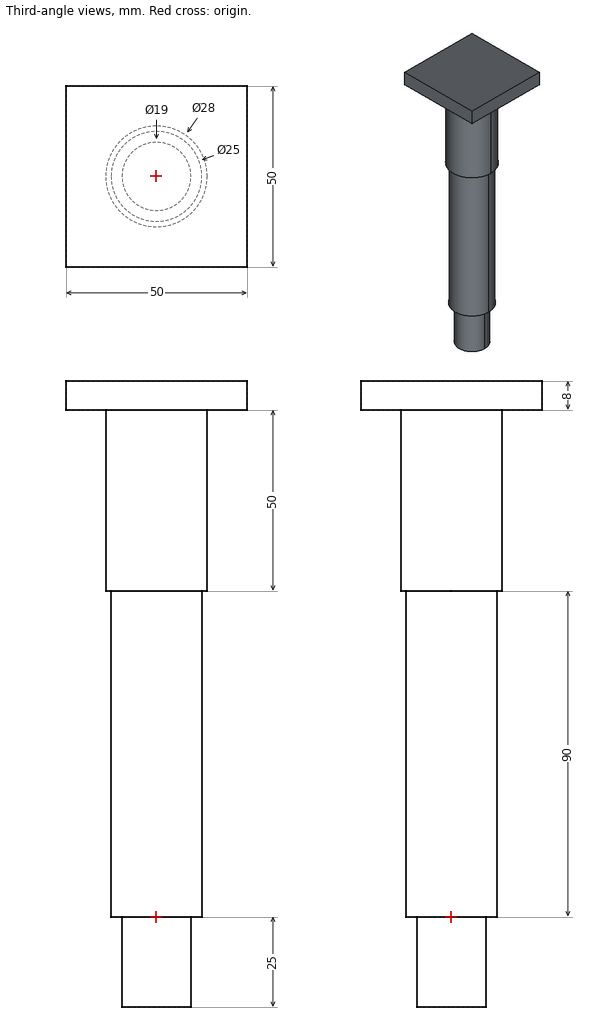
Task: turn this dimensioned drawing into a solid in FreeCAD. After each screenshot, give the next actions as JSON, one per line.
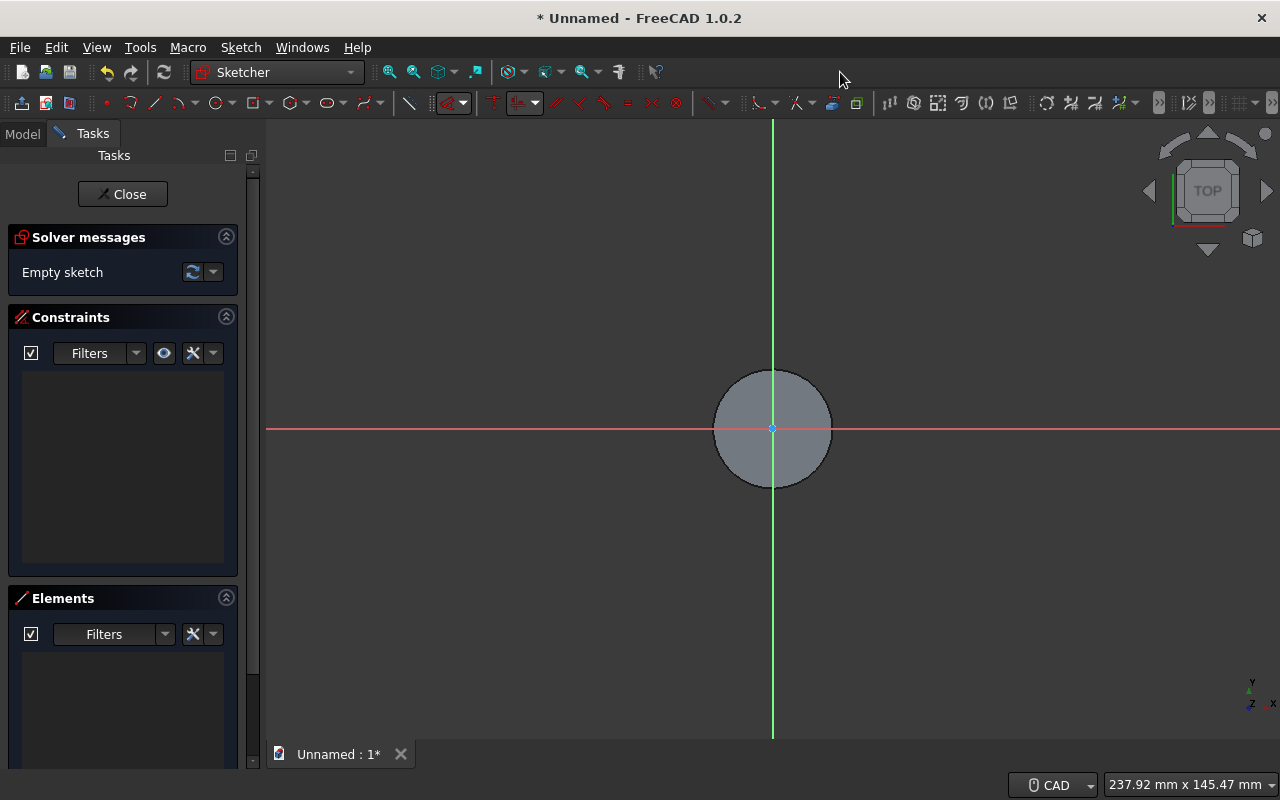
{"action": "scroll", "coordinate": [856, 429], "scroll_direction": "up", "scroll_amount": 3}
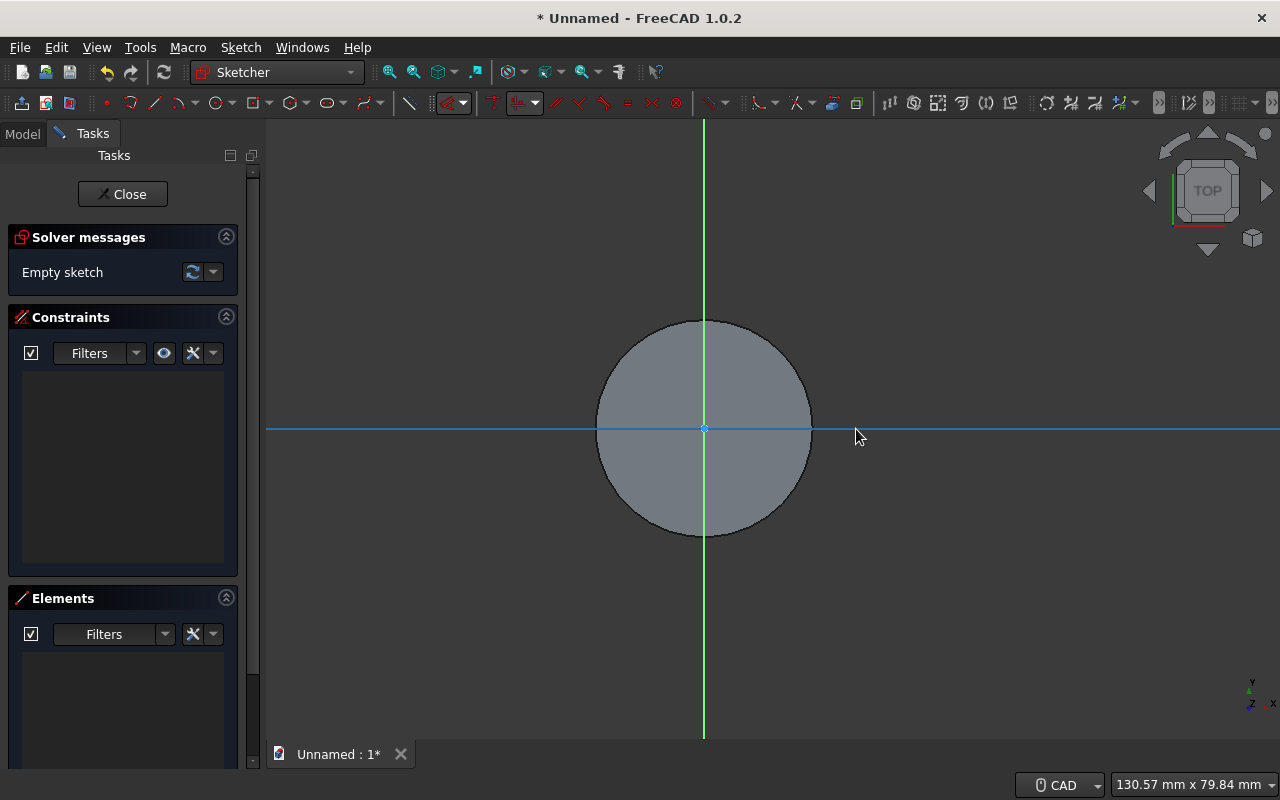
{"action": "key", "text": "g v"}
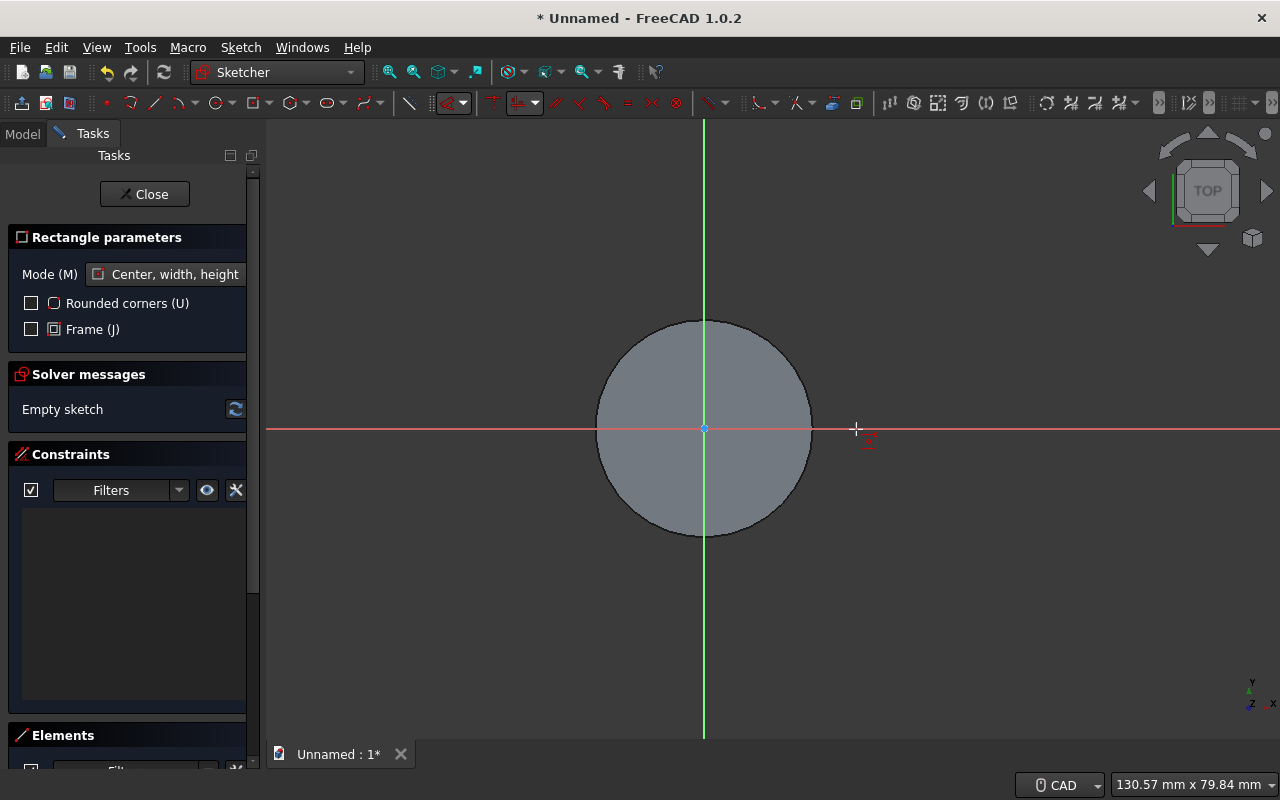
{"action": "left_click", "coordinate": [704, 429]}
{"action": "left_click", "coordinate": [898, 234]}
{"action": "key", "text": "Escape"}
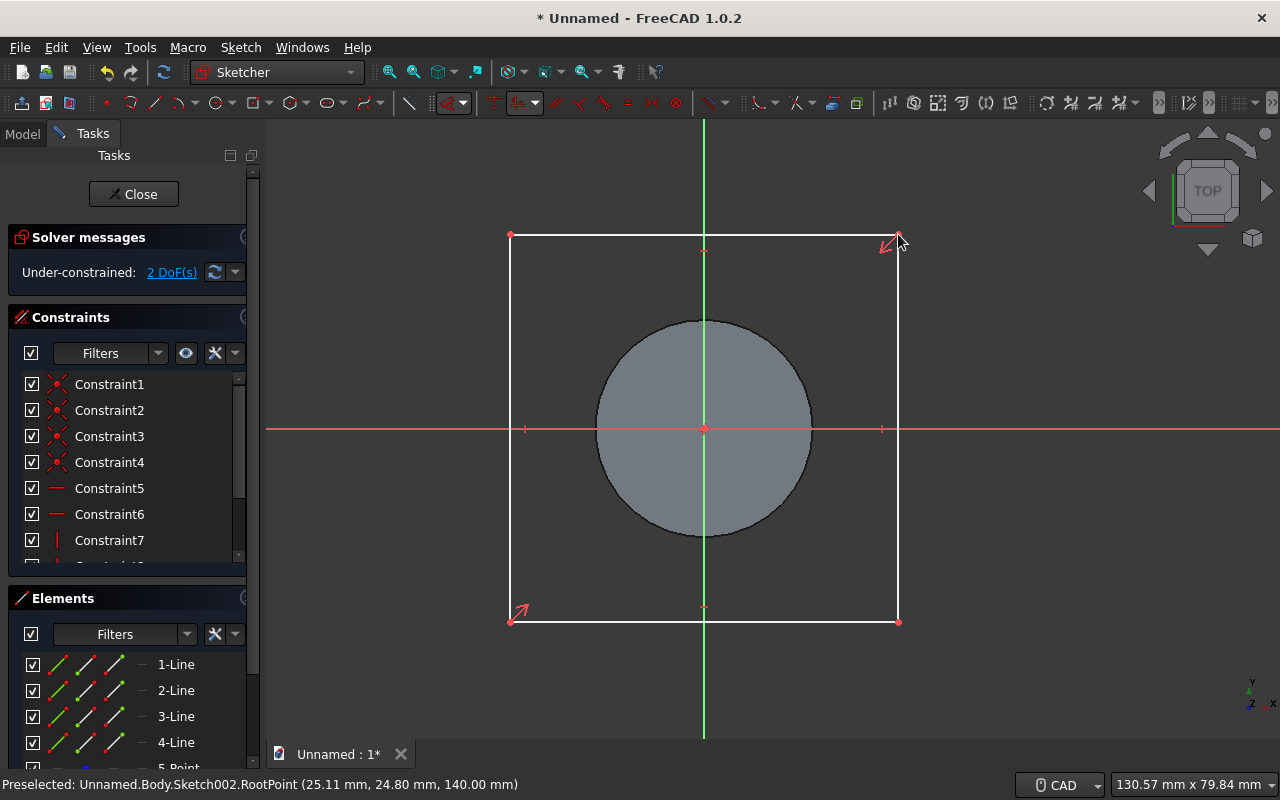
{"action": "left_click", "coordinate": [448, 104]}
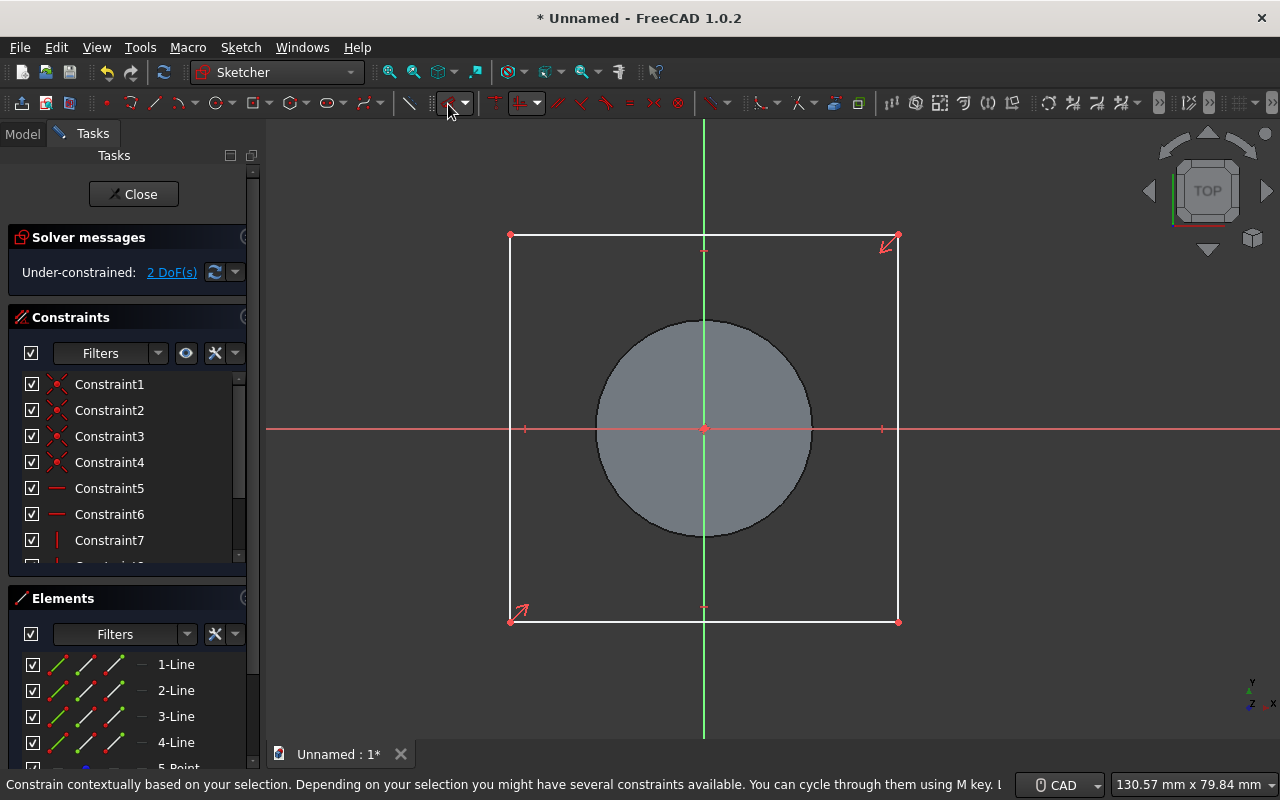
{"action": "left_click", "coordinate": [626, 622]}
{"action": "left_click", "coordinate": [615, 656]}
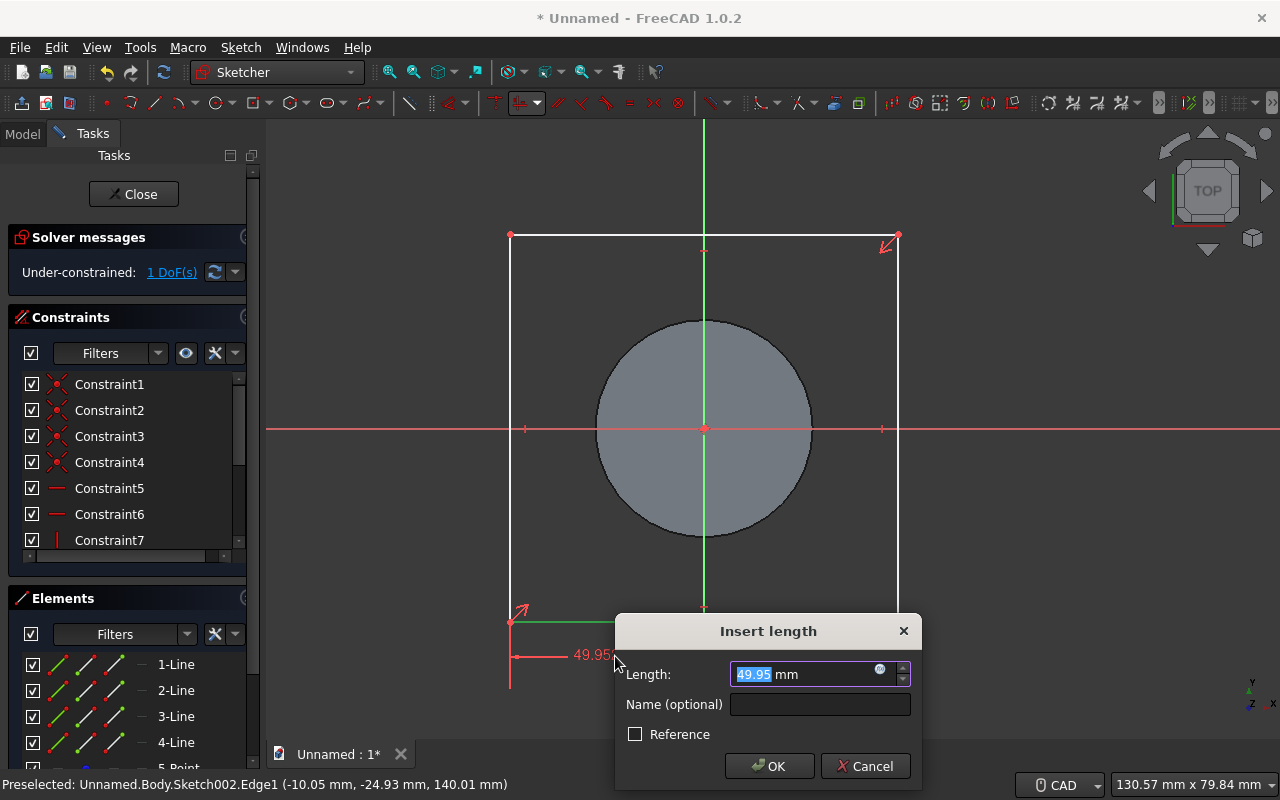
{"action": "type", "text": "50"}
{"action": "key", "text": "Return"}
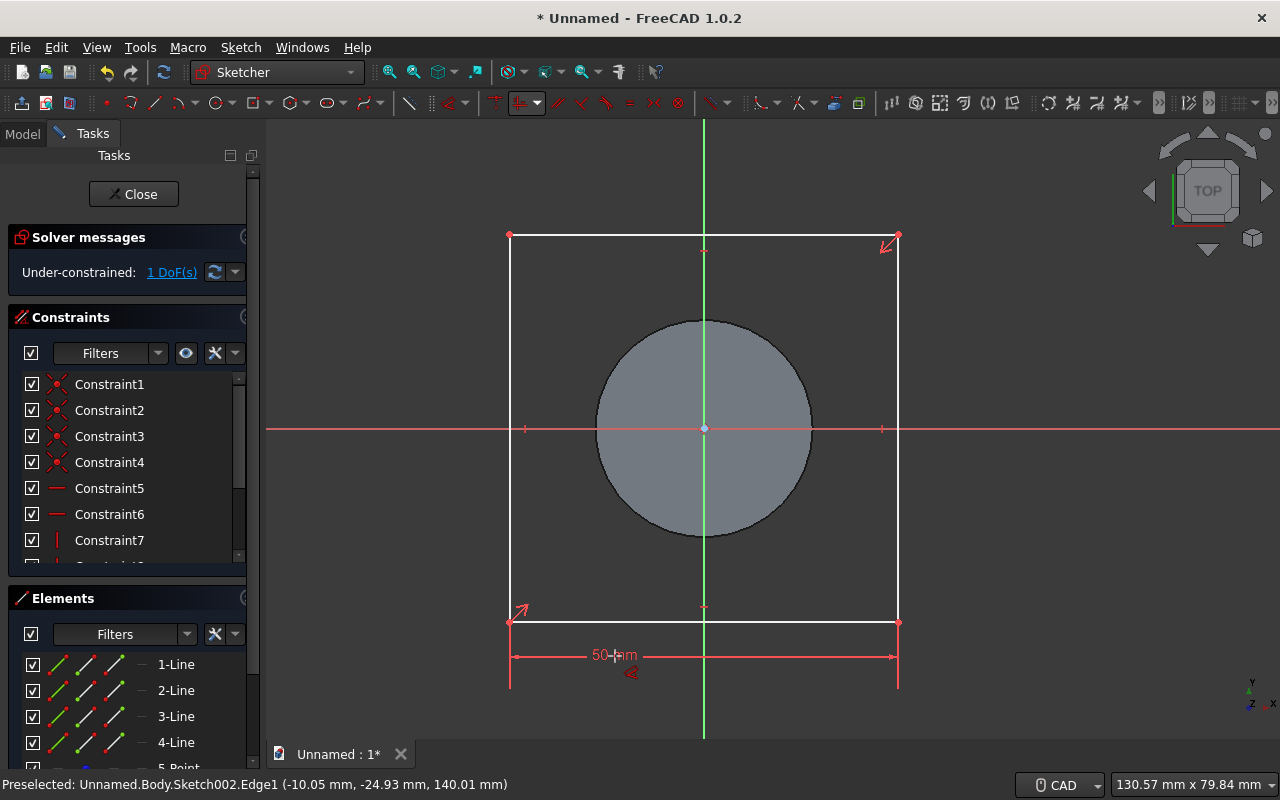
{"action": "left_click", "coordinate": [898, 506]}
{"action": "left_click", "coordinate": [932, 340]}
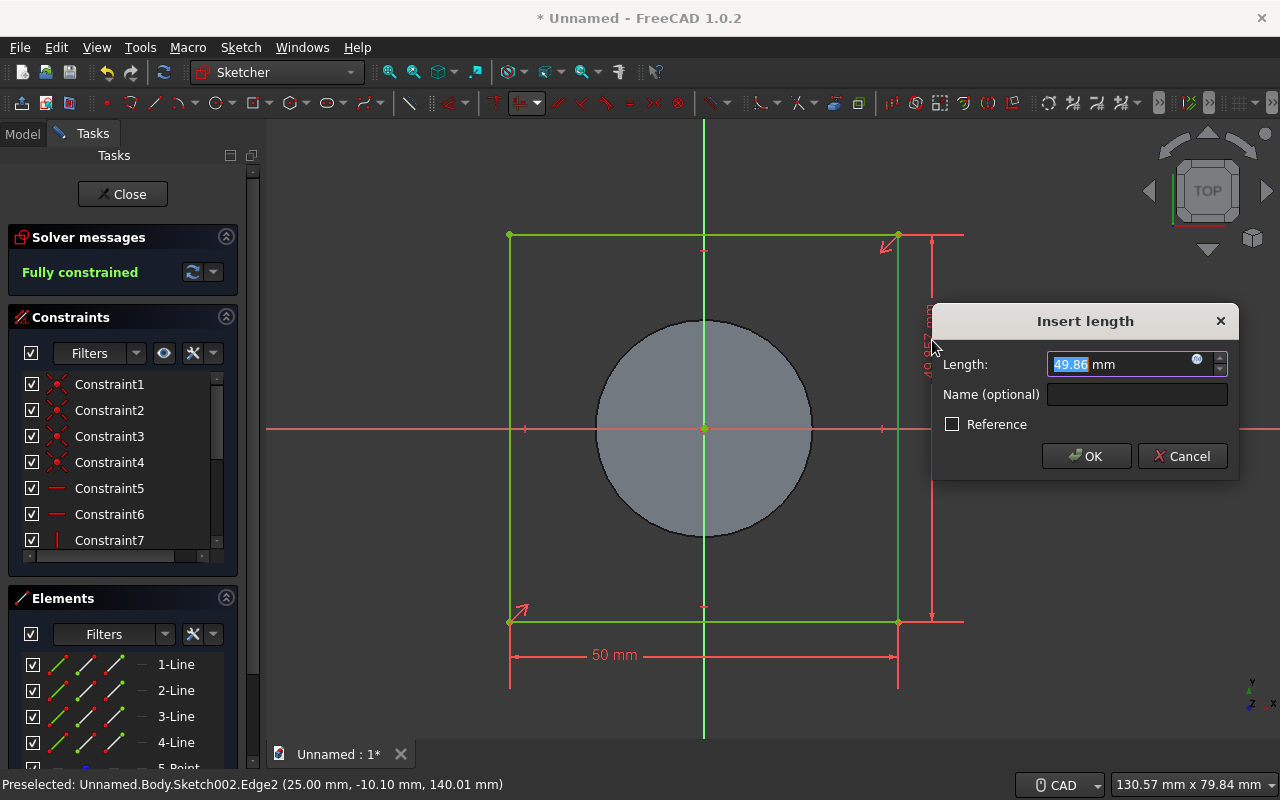
{"action": "type", "text": "50"}
{"action": "key", "text": "Return"}
{"action": "key", "text": "Escape"}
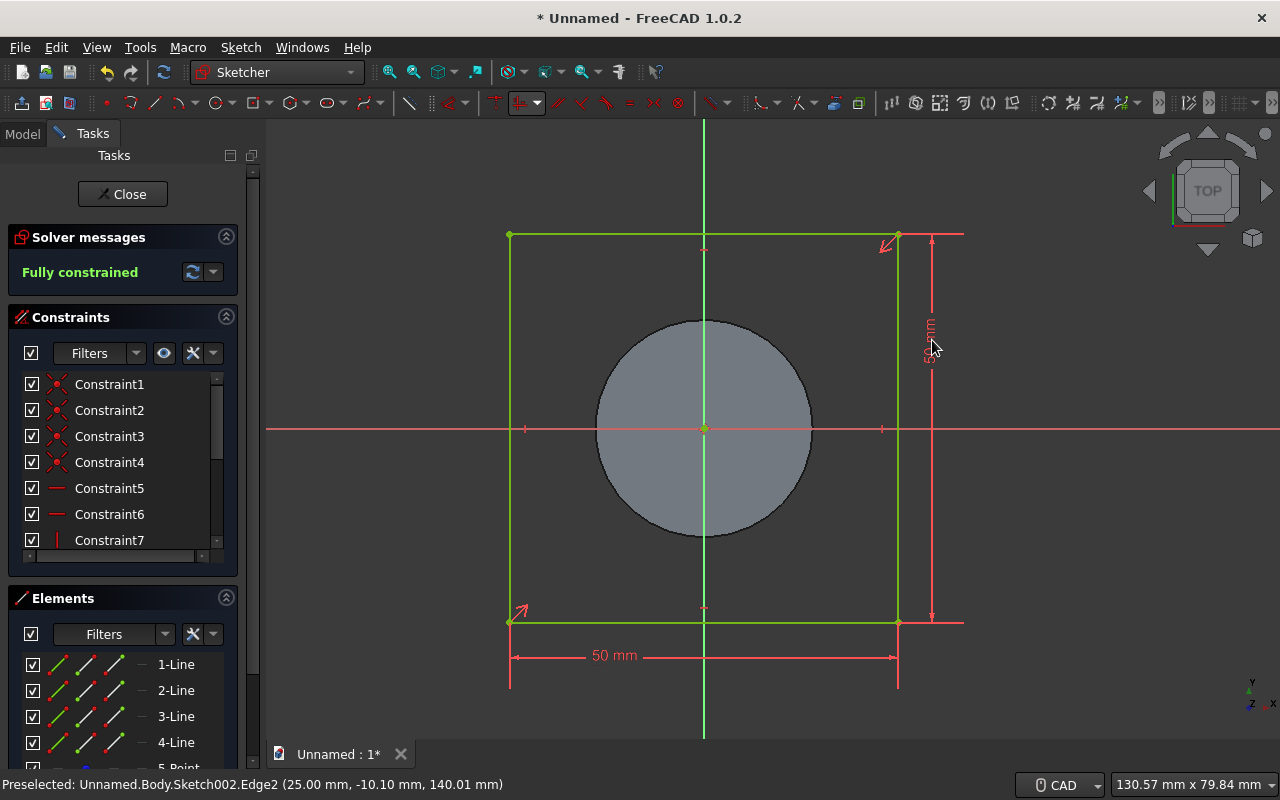
{"action": "left_click", "coordinate": [123, 194]}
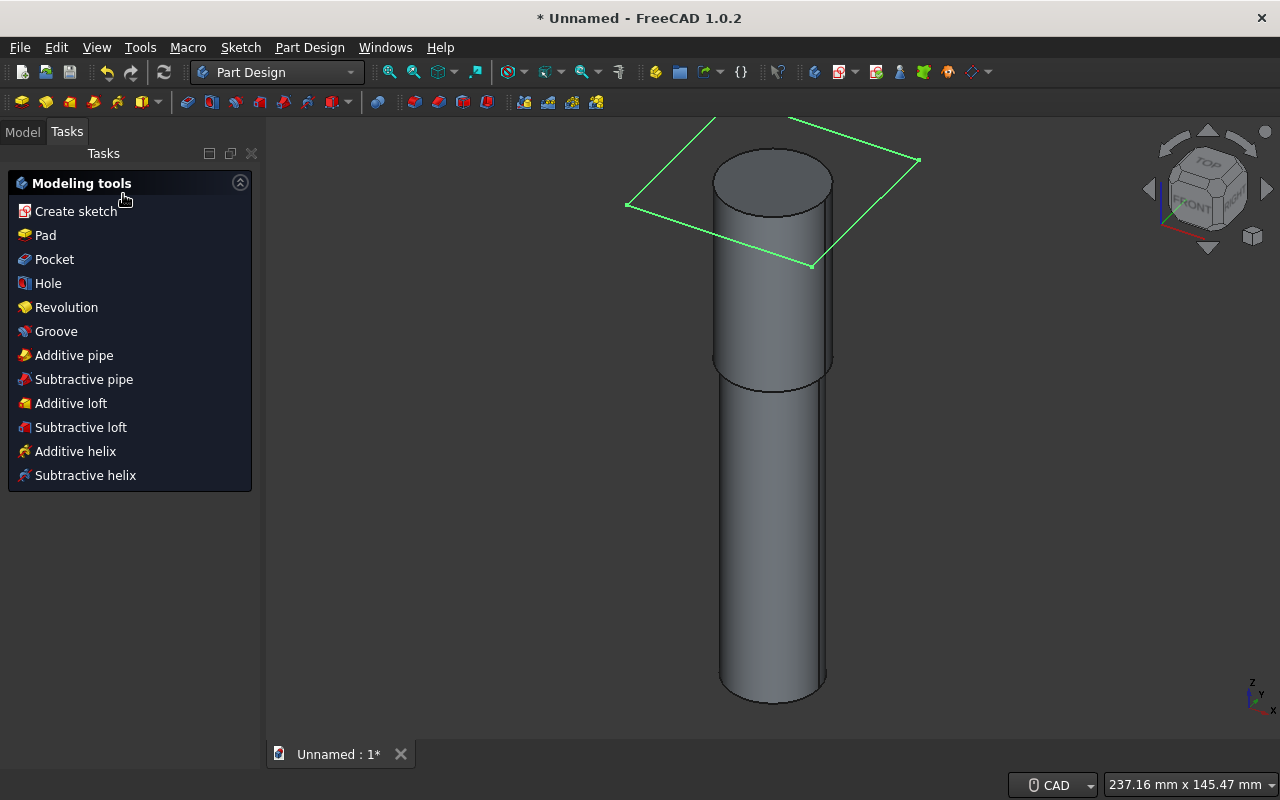
{"action": "left_click", "coordinate": [22, 102]}